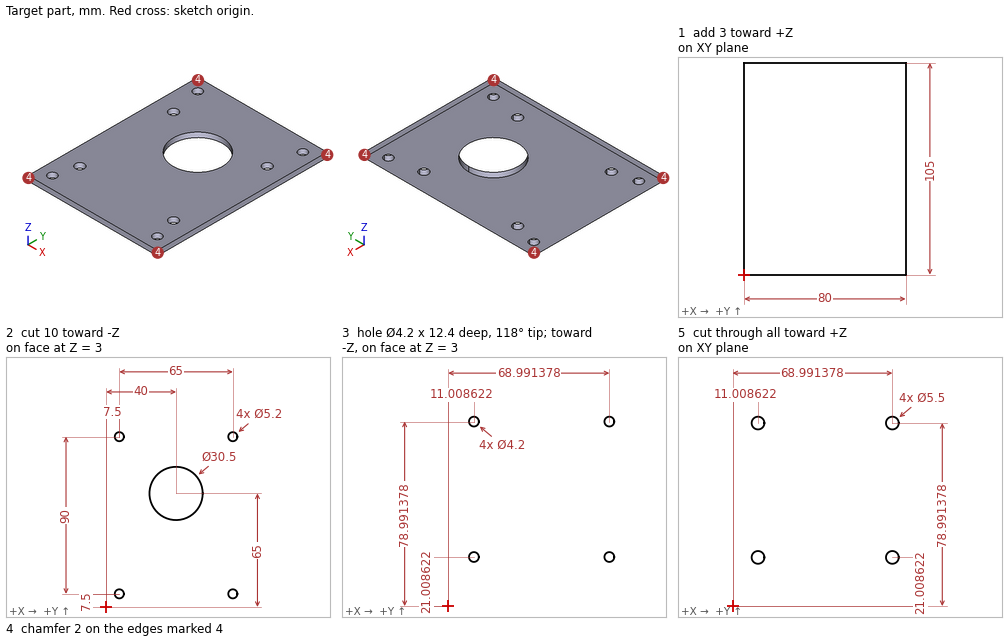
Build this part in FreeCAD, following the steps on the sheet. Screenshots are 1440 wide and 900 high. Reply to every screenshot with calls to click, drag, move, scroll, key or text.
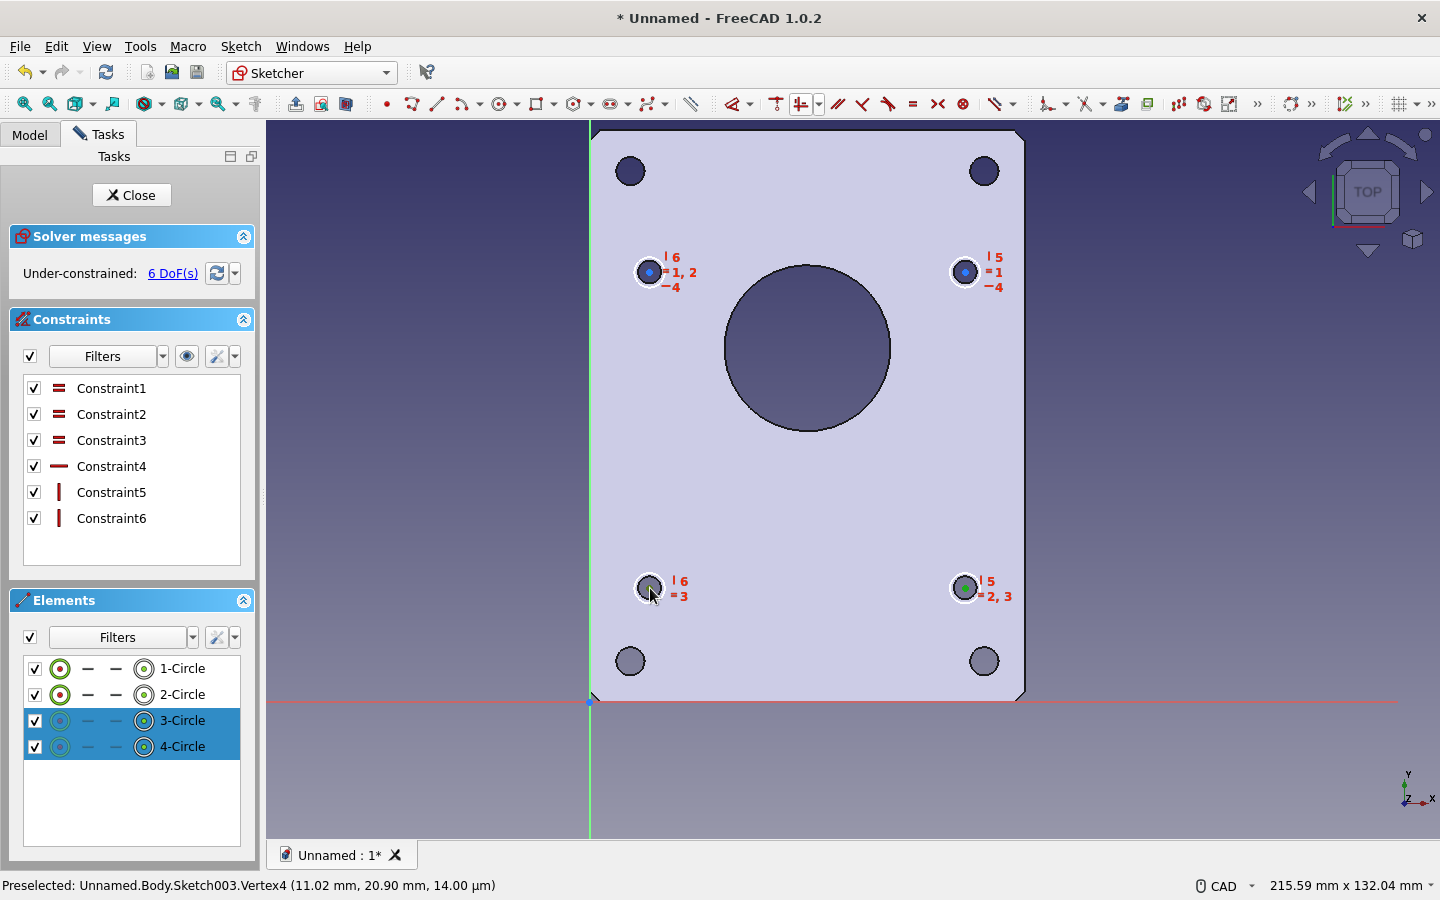
key(h)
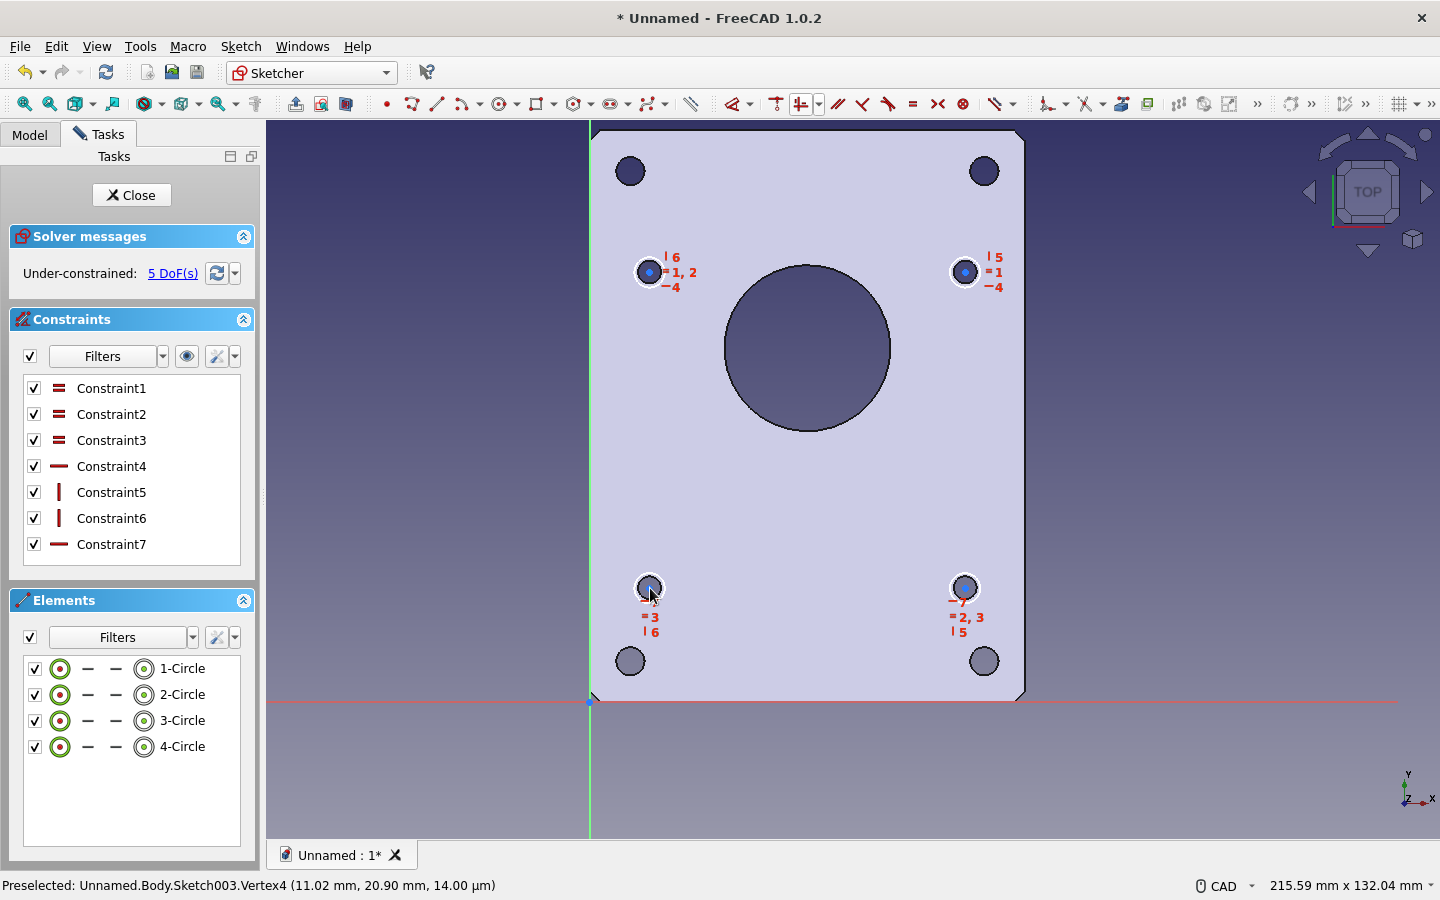
click(732, 104)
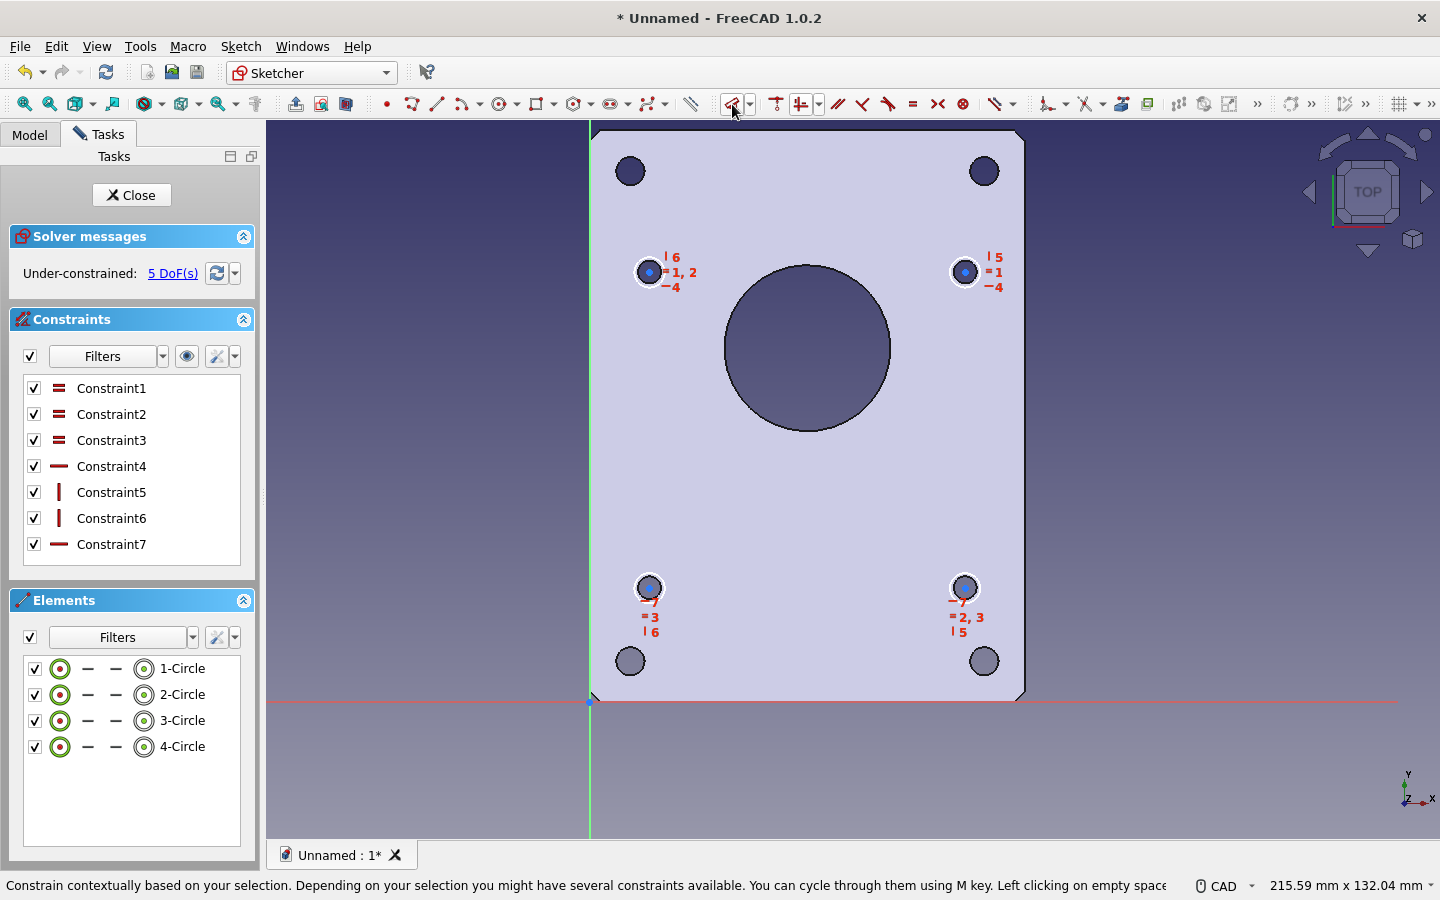
scroll(976, 262, up, 2)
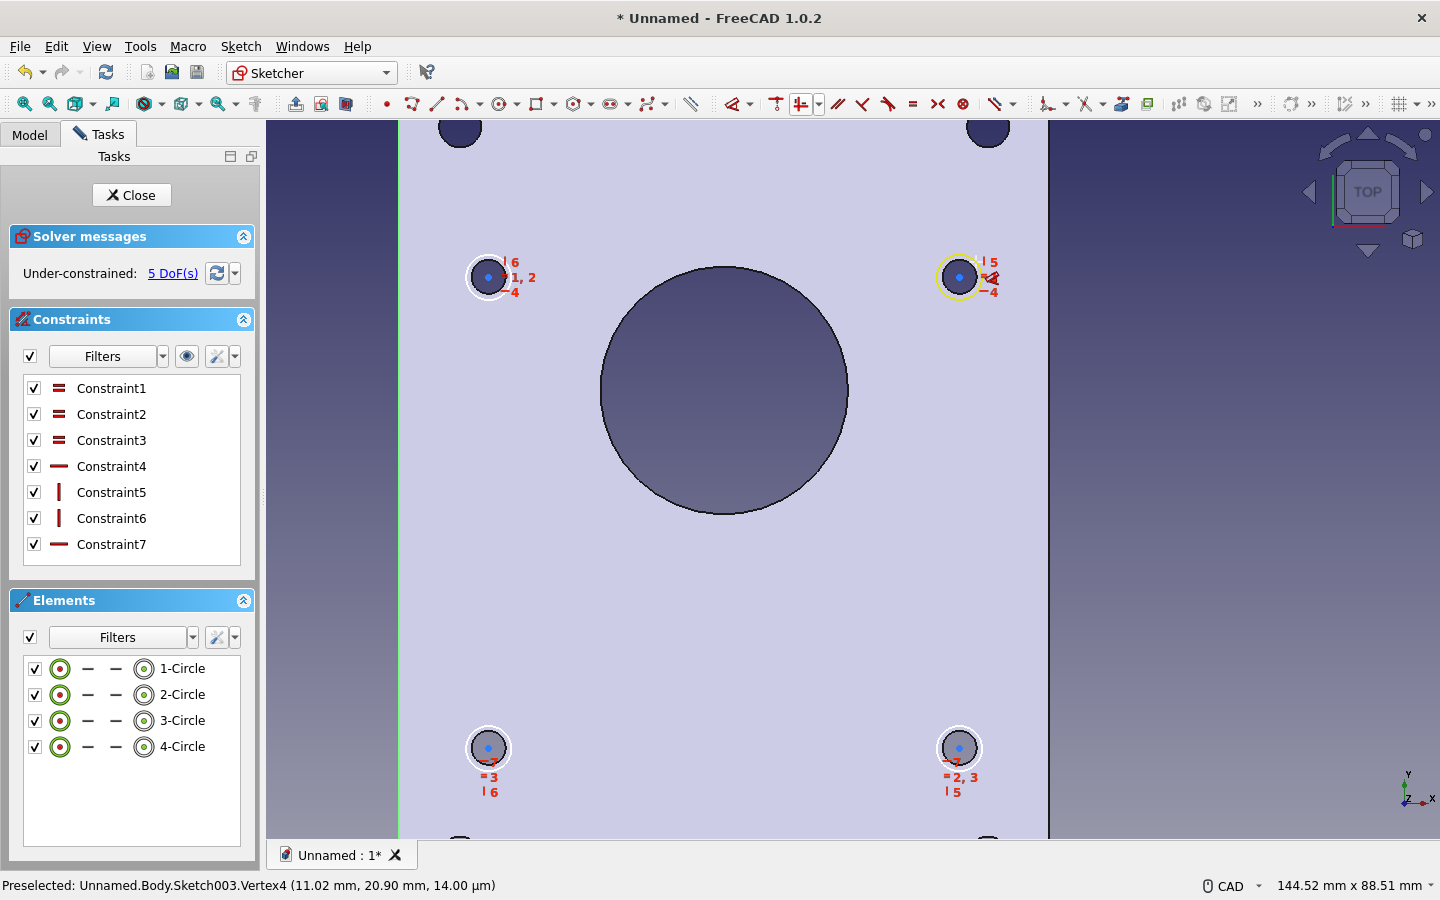
click(975, 261)
click(997, 238)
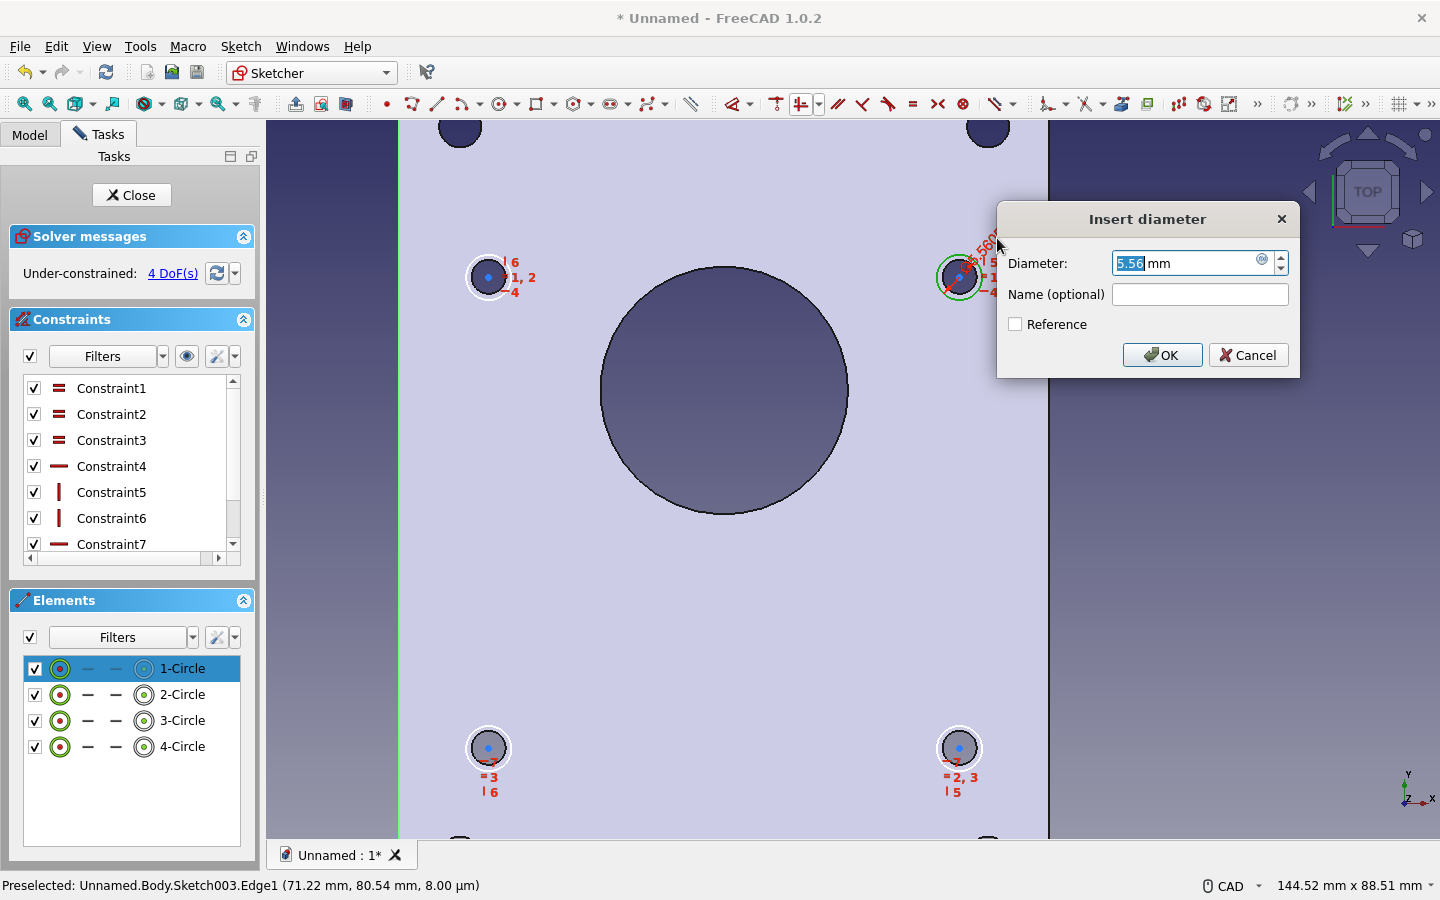
text(5.5)
key(Return)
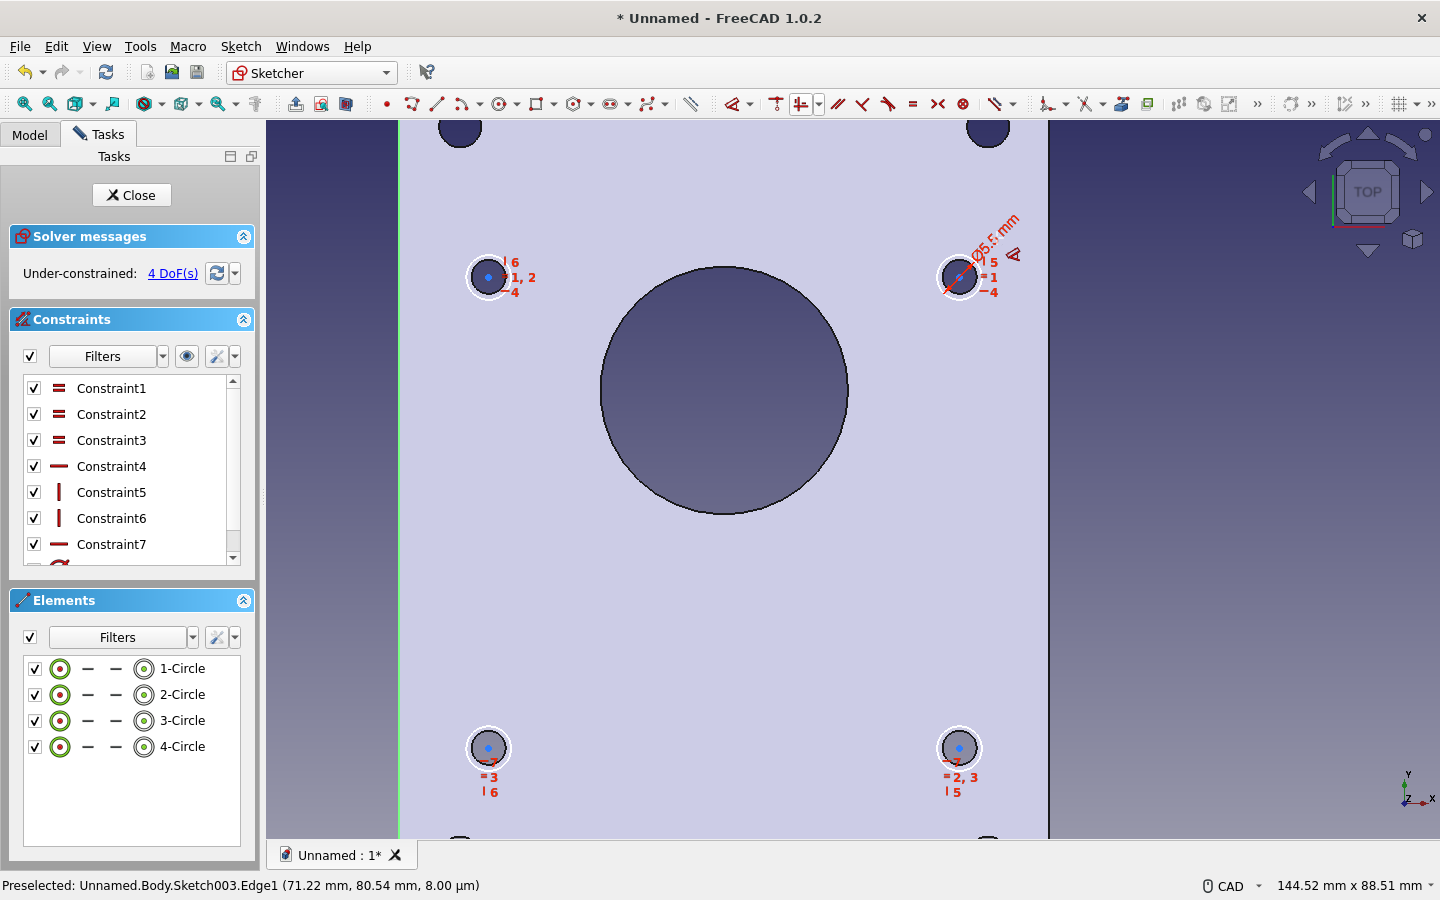
click(959, 277)
click(679, 243)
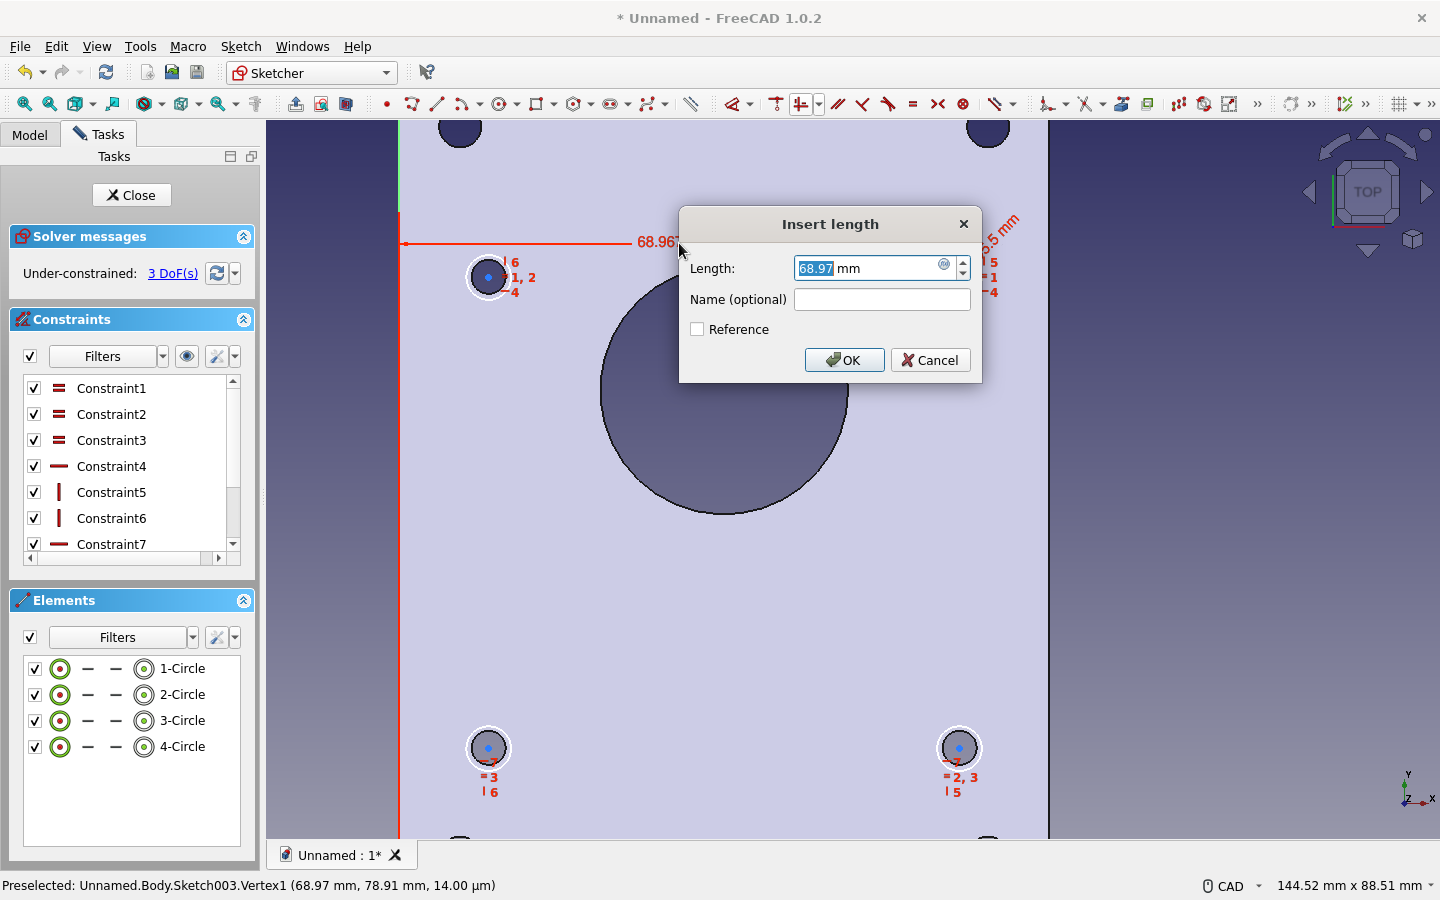
text(68.991378)
key(Return)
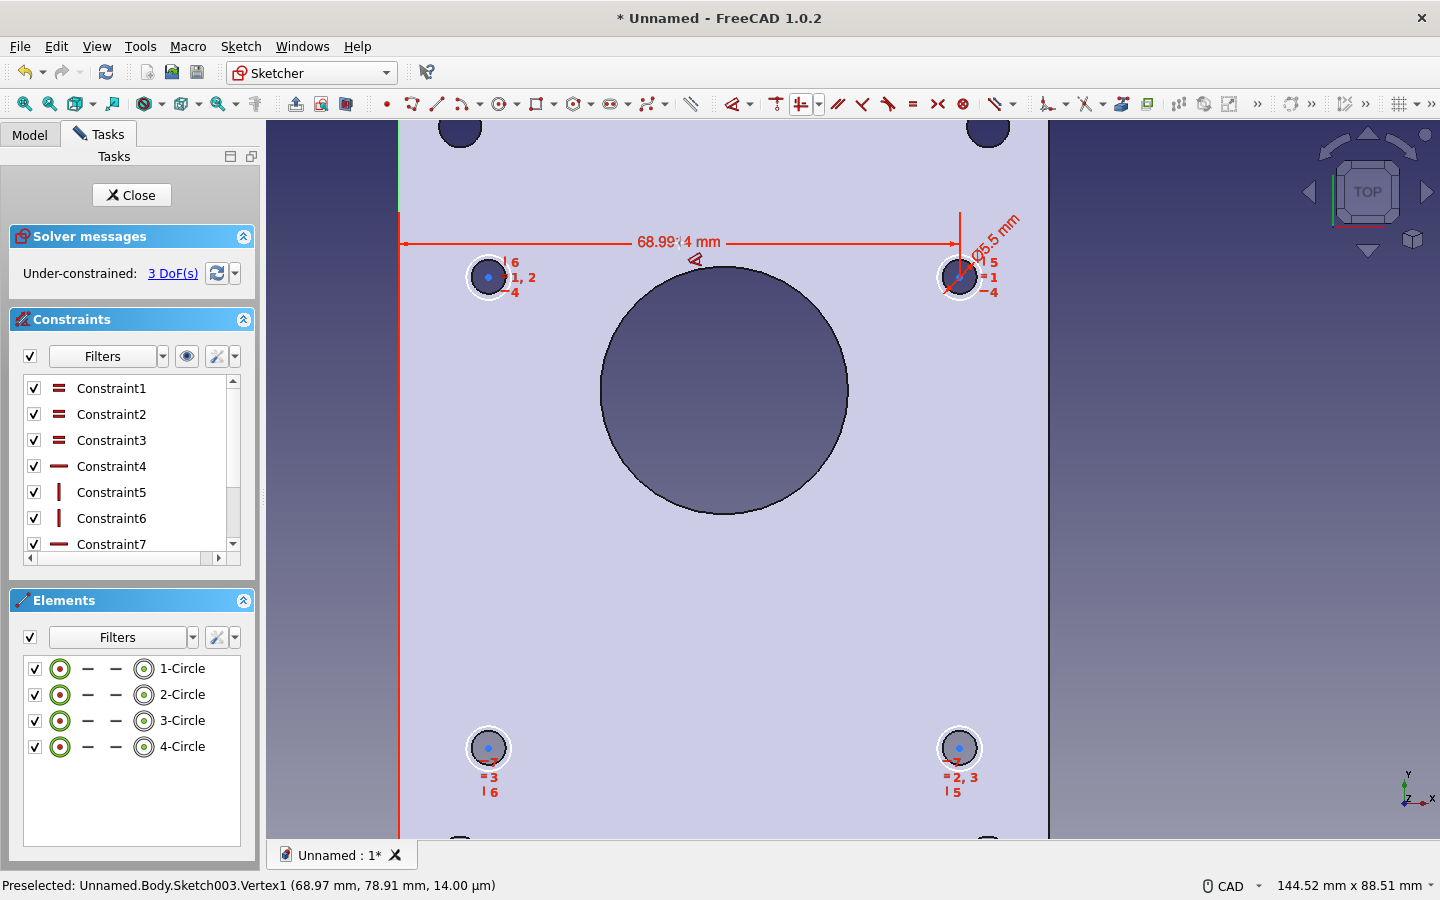
click(960, 277)
click(365, 544)